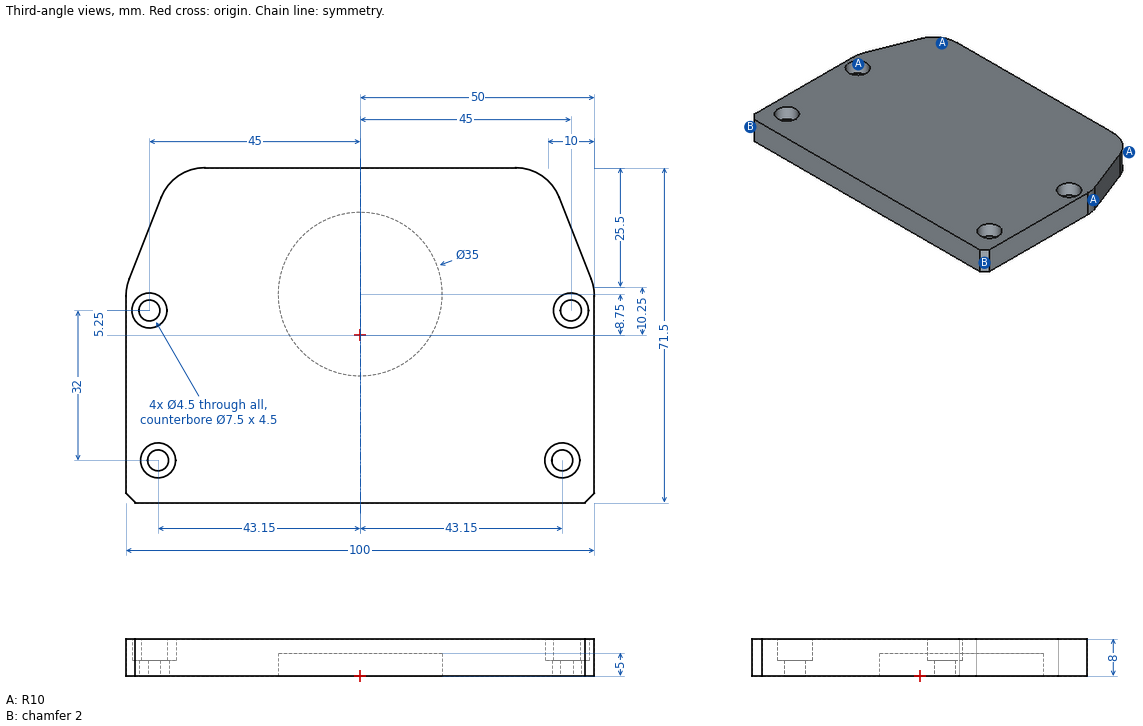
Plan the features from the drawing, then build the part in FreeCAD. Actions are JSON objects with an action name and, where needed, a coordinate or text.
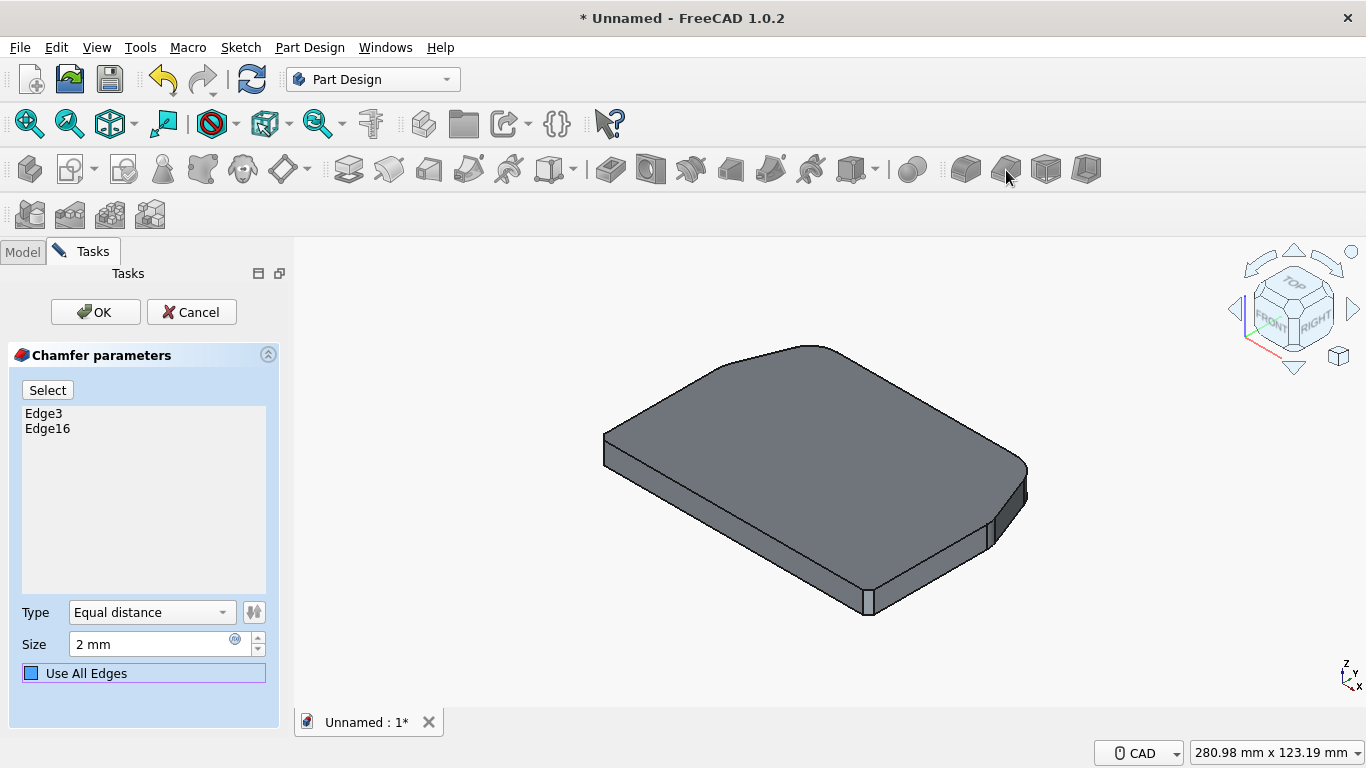
{"action": "left_click", "coordinate": [96, 312]}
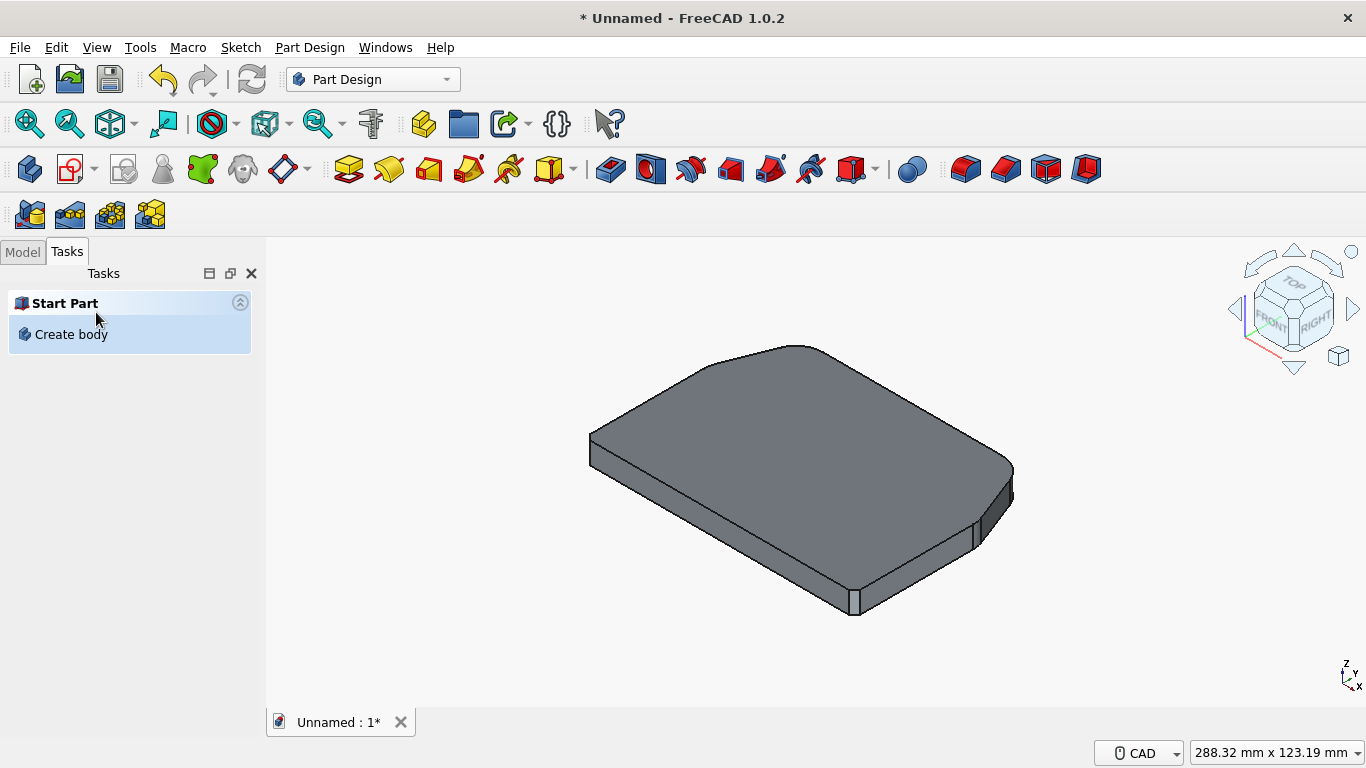
{"action": "left_click", "coordinate": [70, 170]}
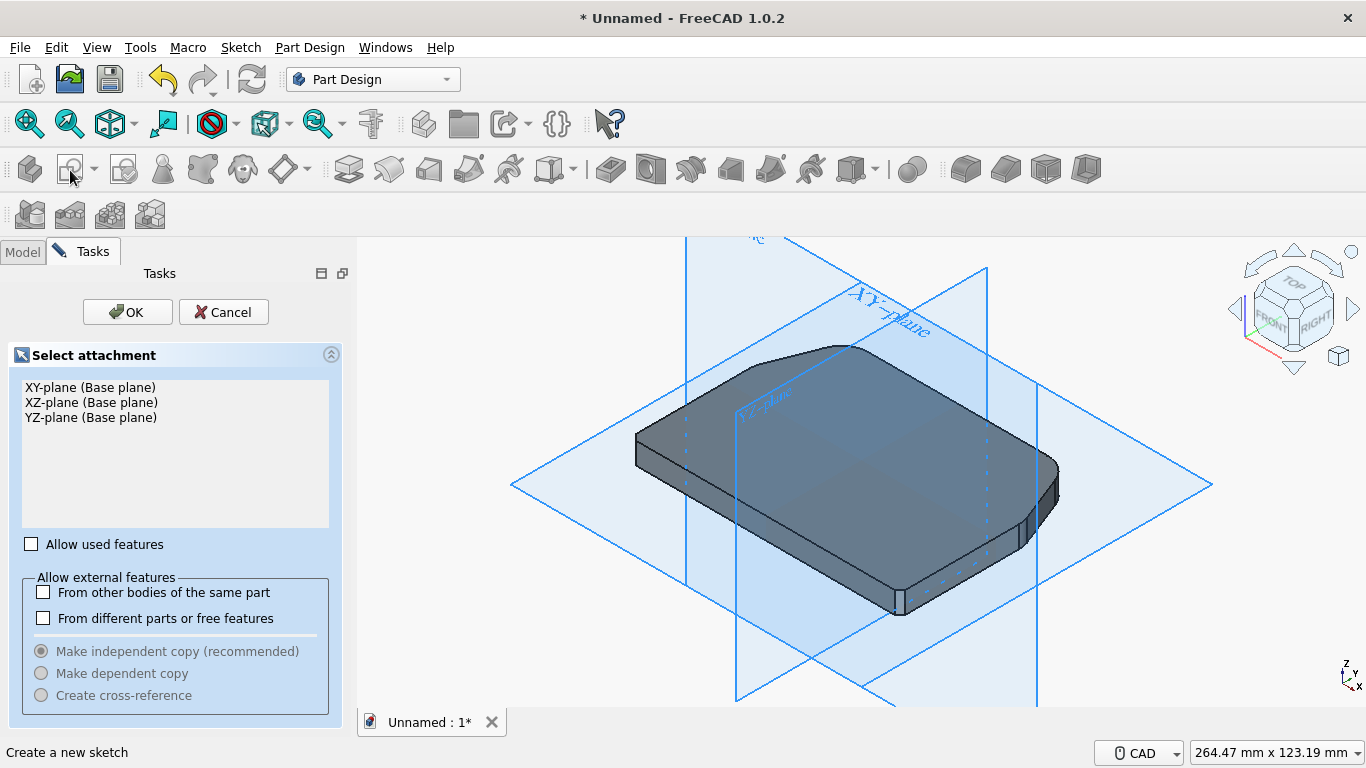
{"action": "left_click", "coordinate": [82, 388]}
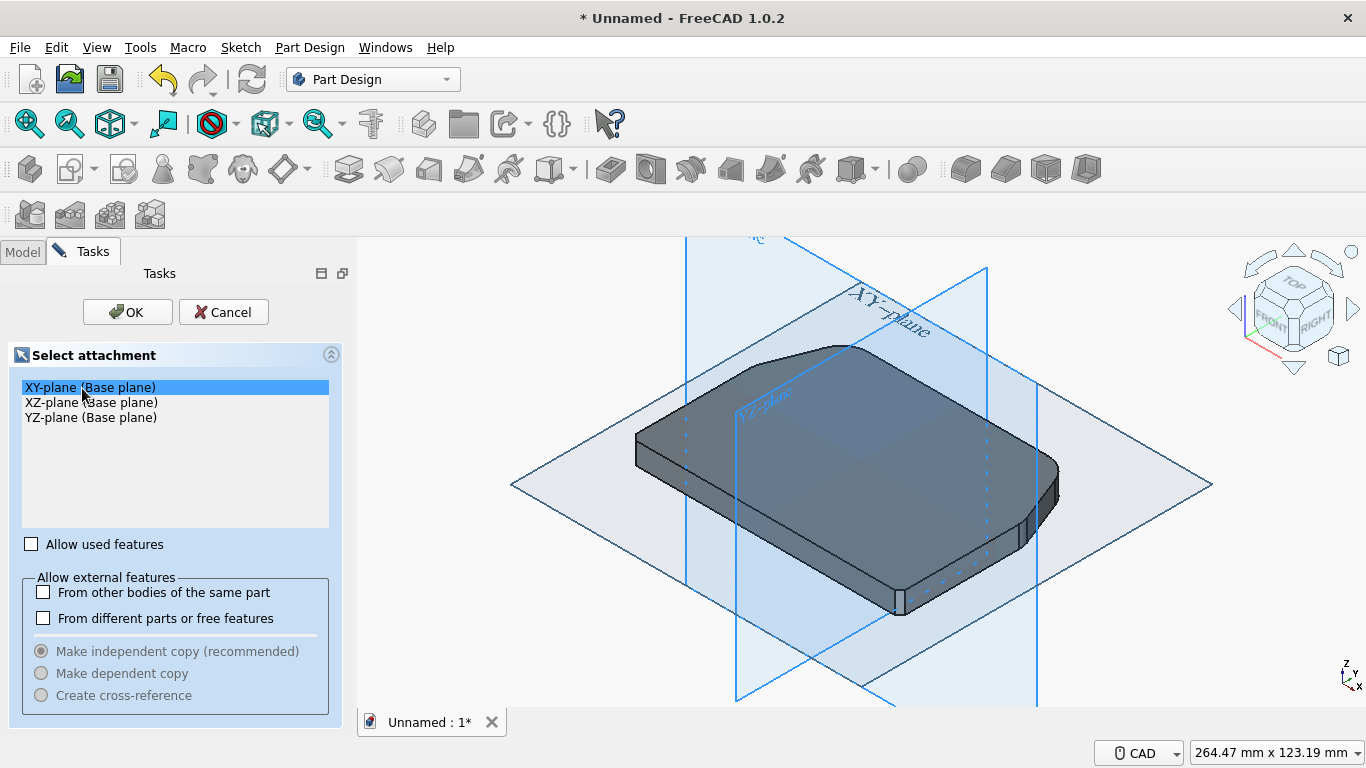
{"action": "left_click", "coordinate": [128, 312]}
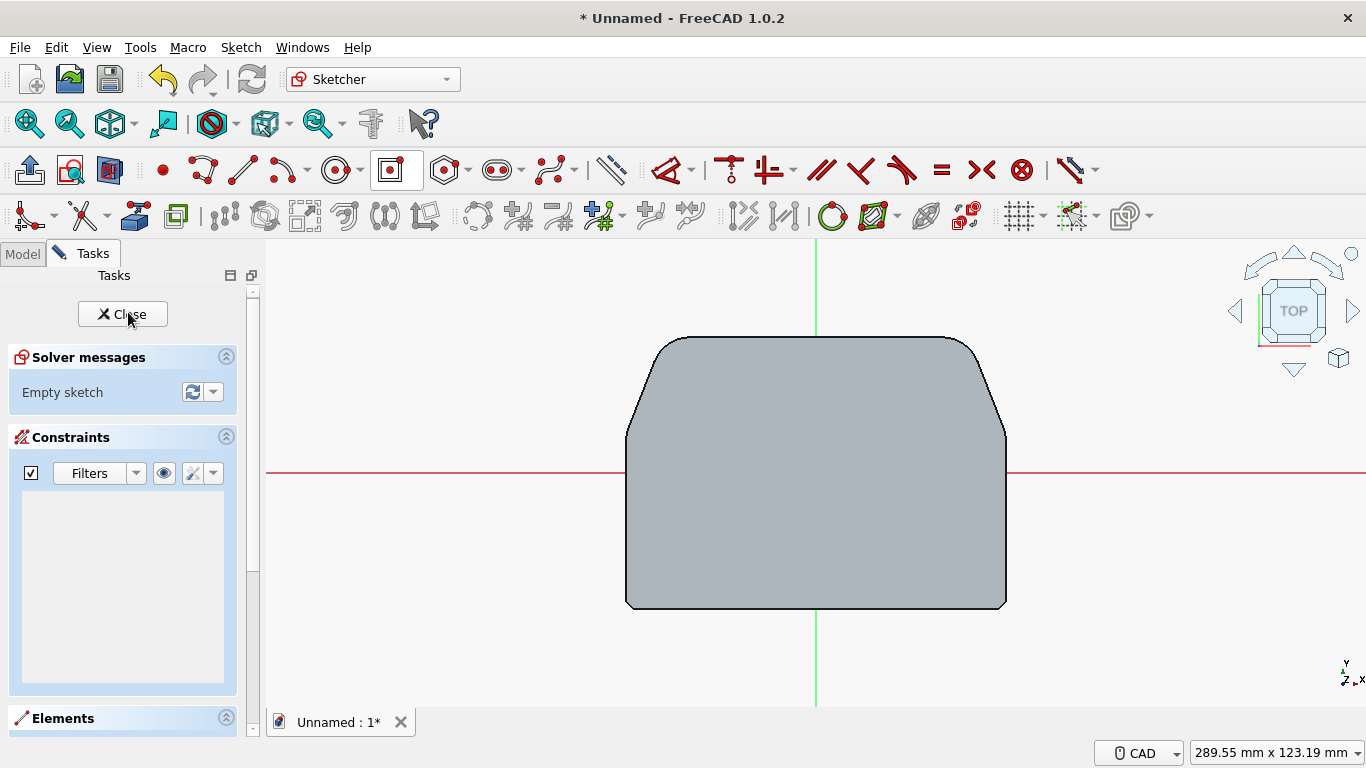
{"action": "left_click", "coordinate": [110, 170]}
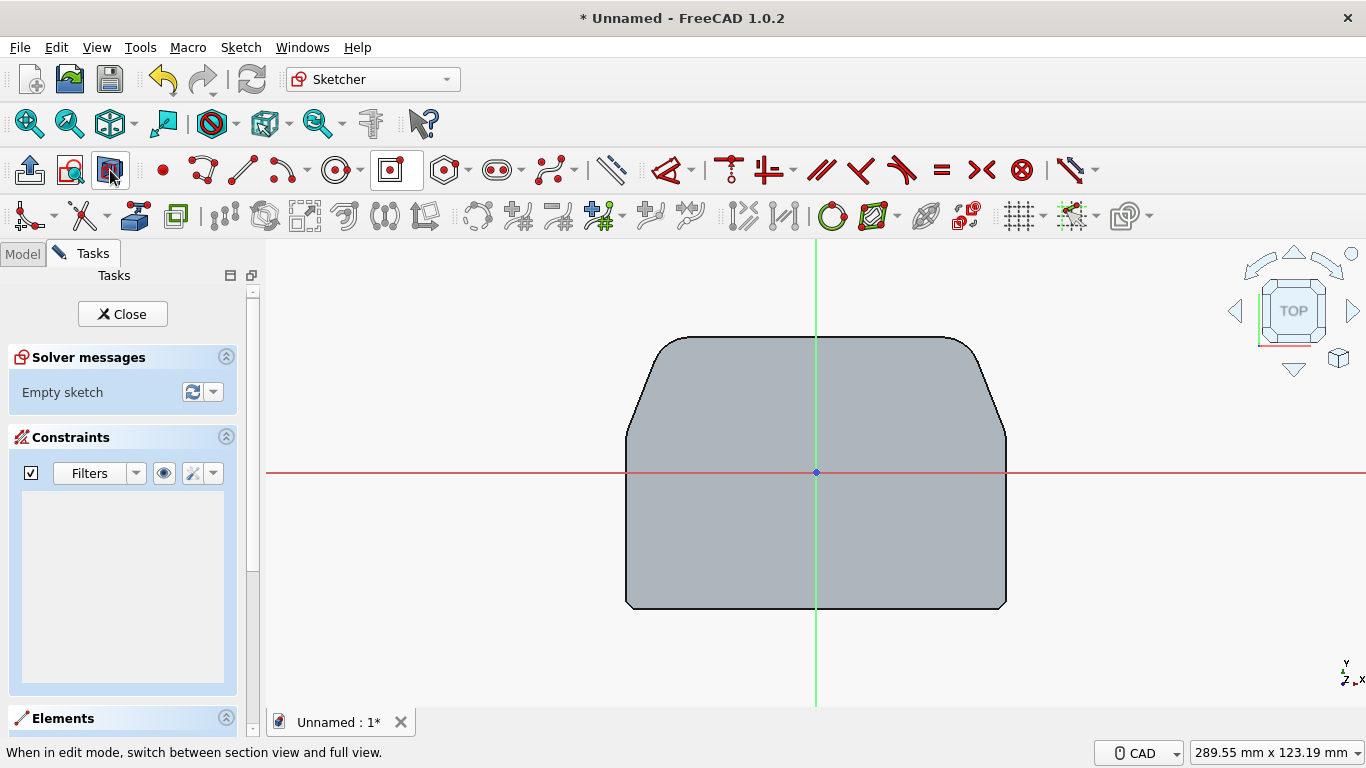
{"action": "scroll", "coordinate": [872, 413], "scroll_direction": "up", "scroll_amount": 4}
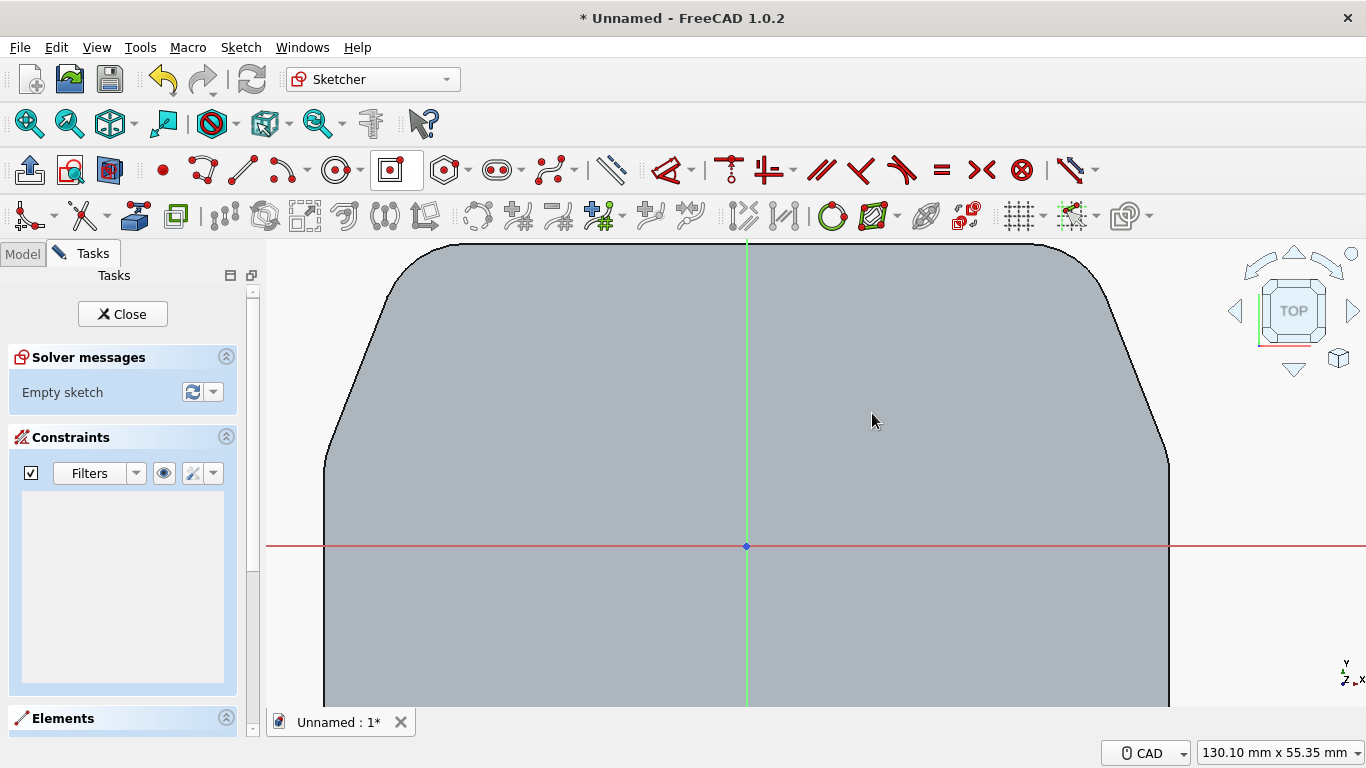
{"action": "left_click", "coordinate": [336, 170]}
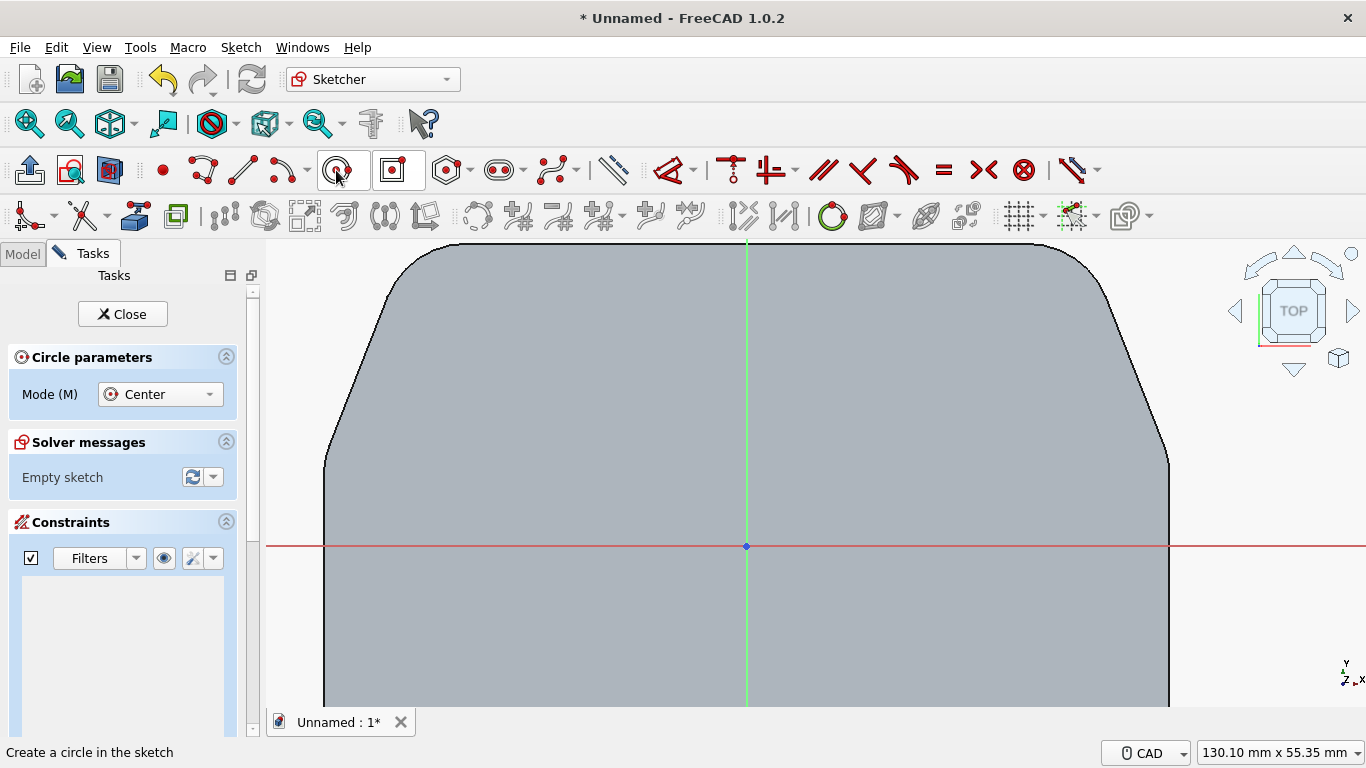
{"action": "left_click", "coordinate": [747, 472]}
{"action": "left_click", "coordinate": [851, 367]}
{"action": "key", "text": "Escape"}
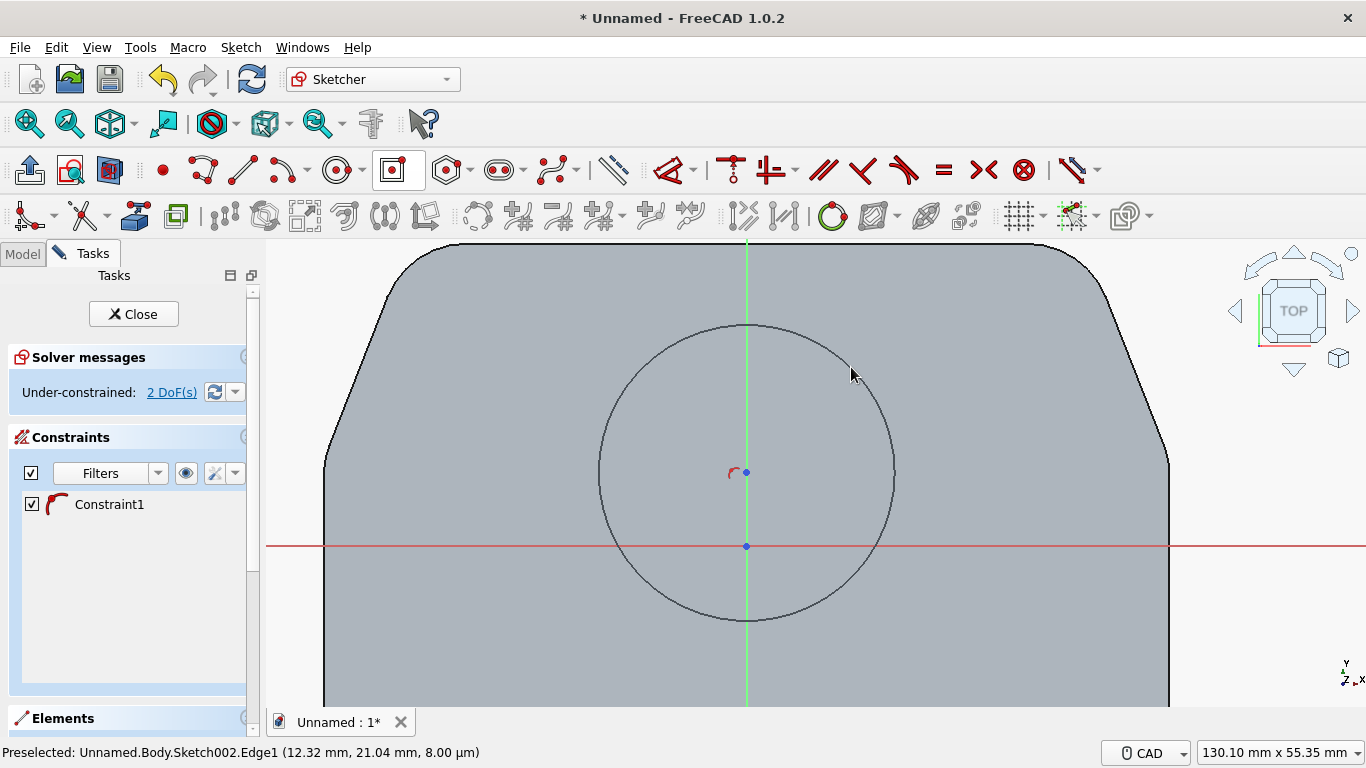
{"action": "left_click", "coordinate": [668, 170]}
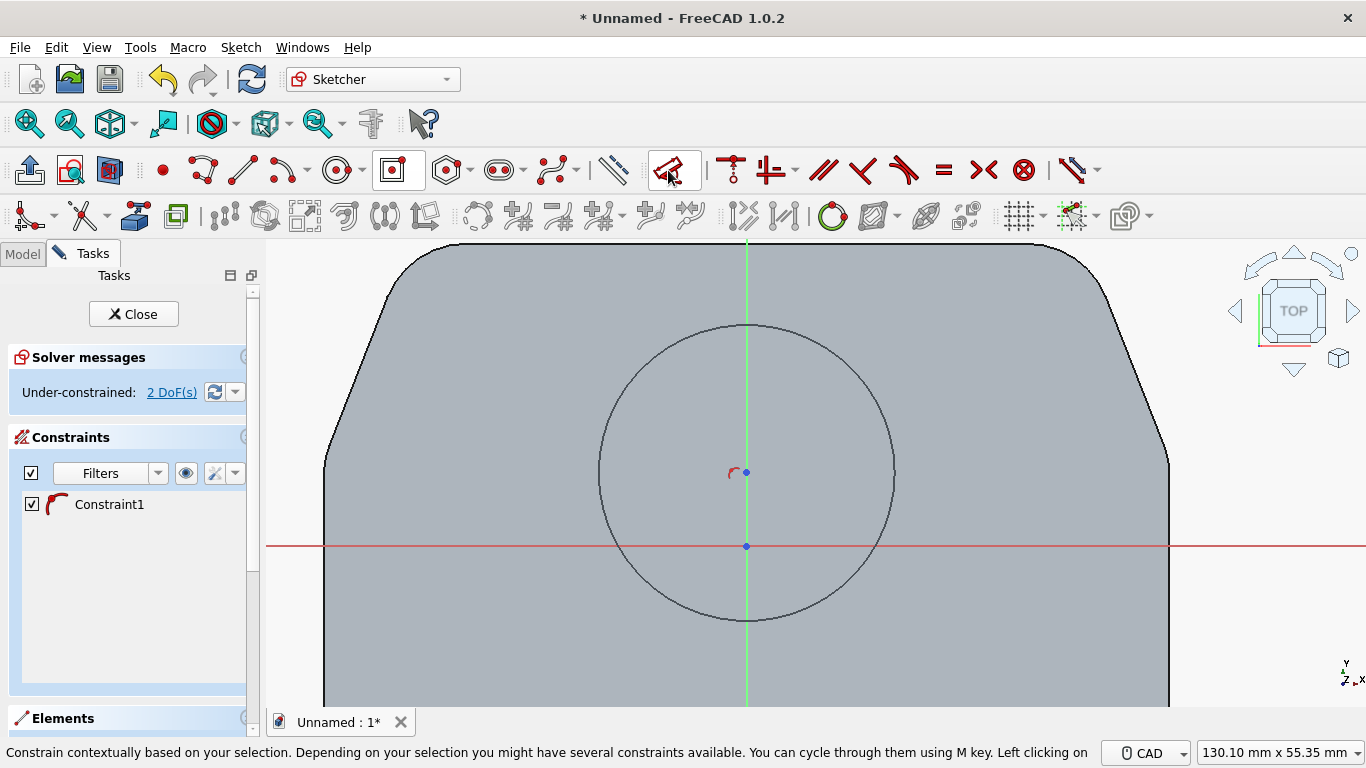
{"action": "left_click", "coordinate": [851, 368]}
{"action": "left_click", "coordinate": [874, 345]}